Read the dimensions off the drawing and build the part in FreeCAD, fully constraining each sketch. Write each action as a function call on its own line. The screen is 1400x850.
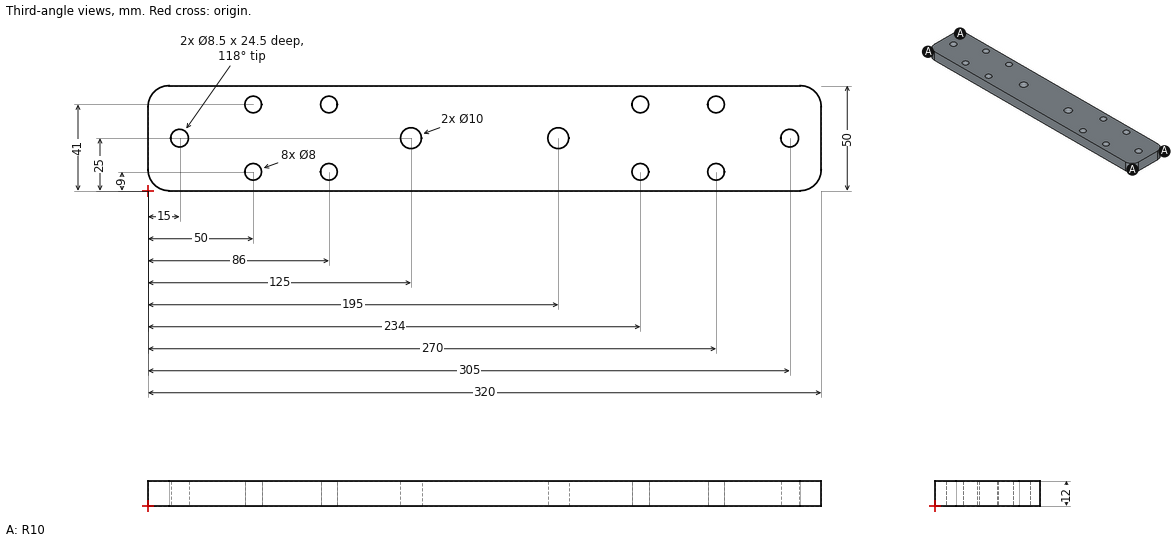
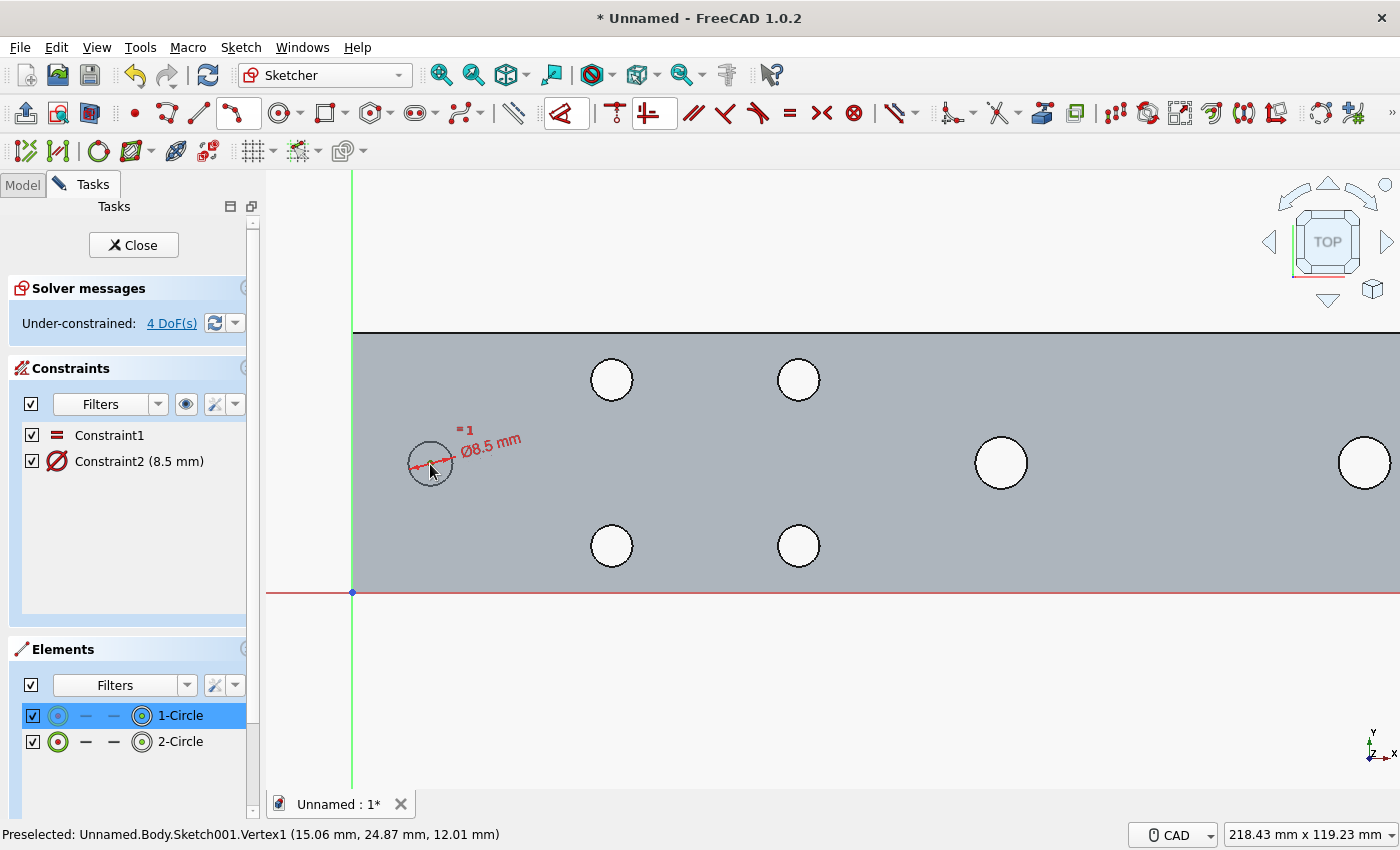
click(584, 114)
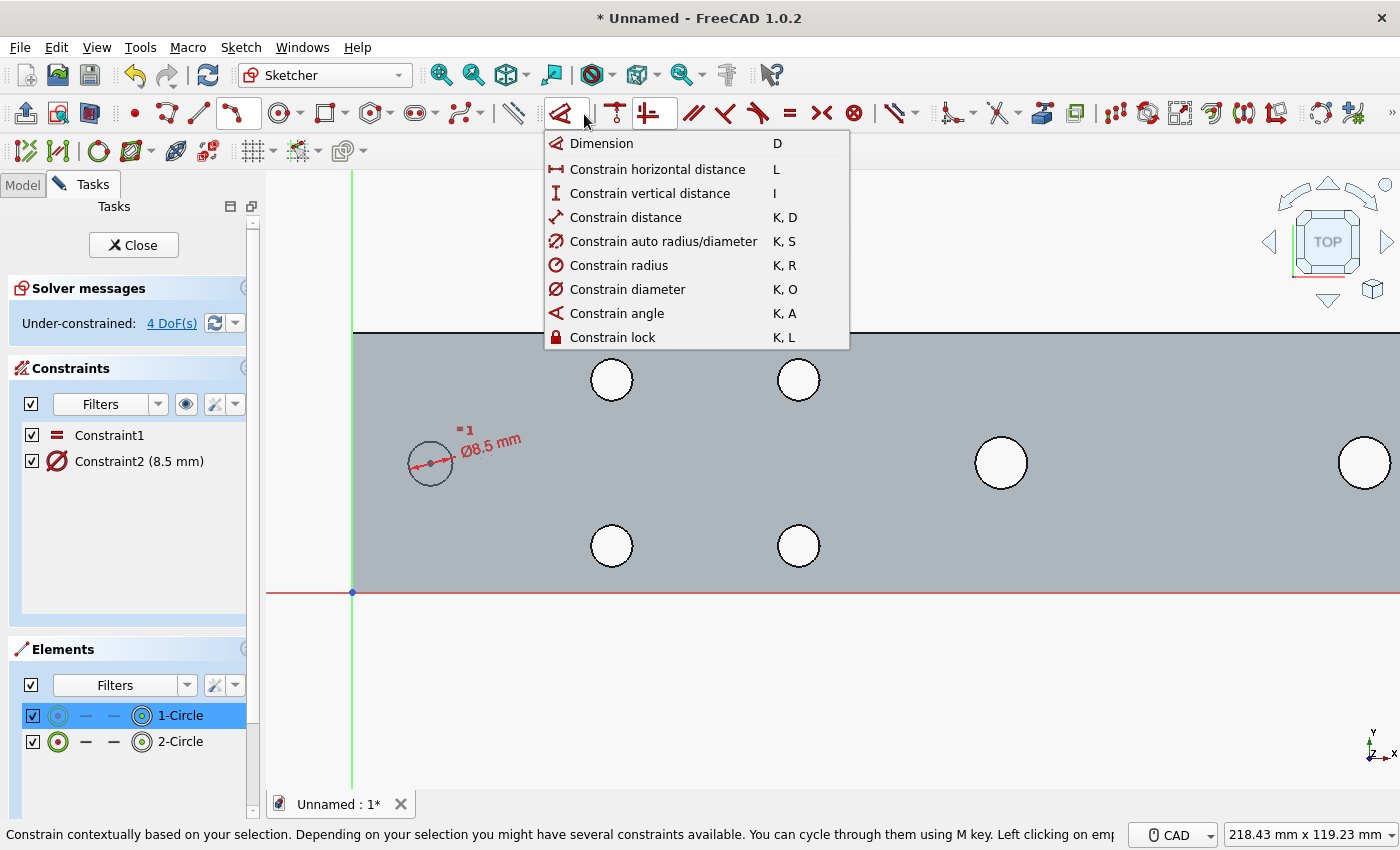
click(697, 169)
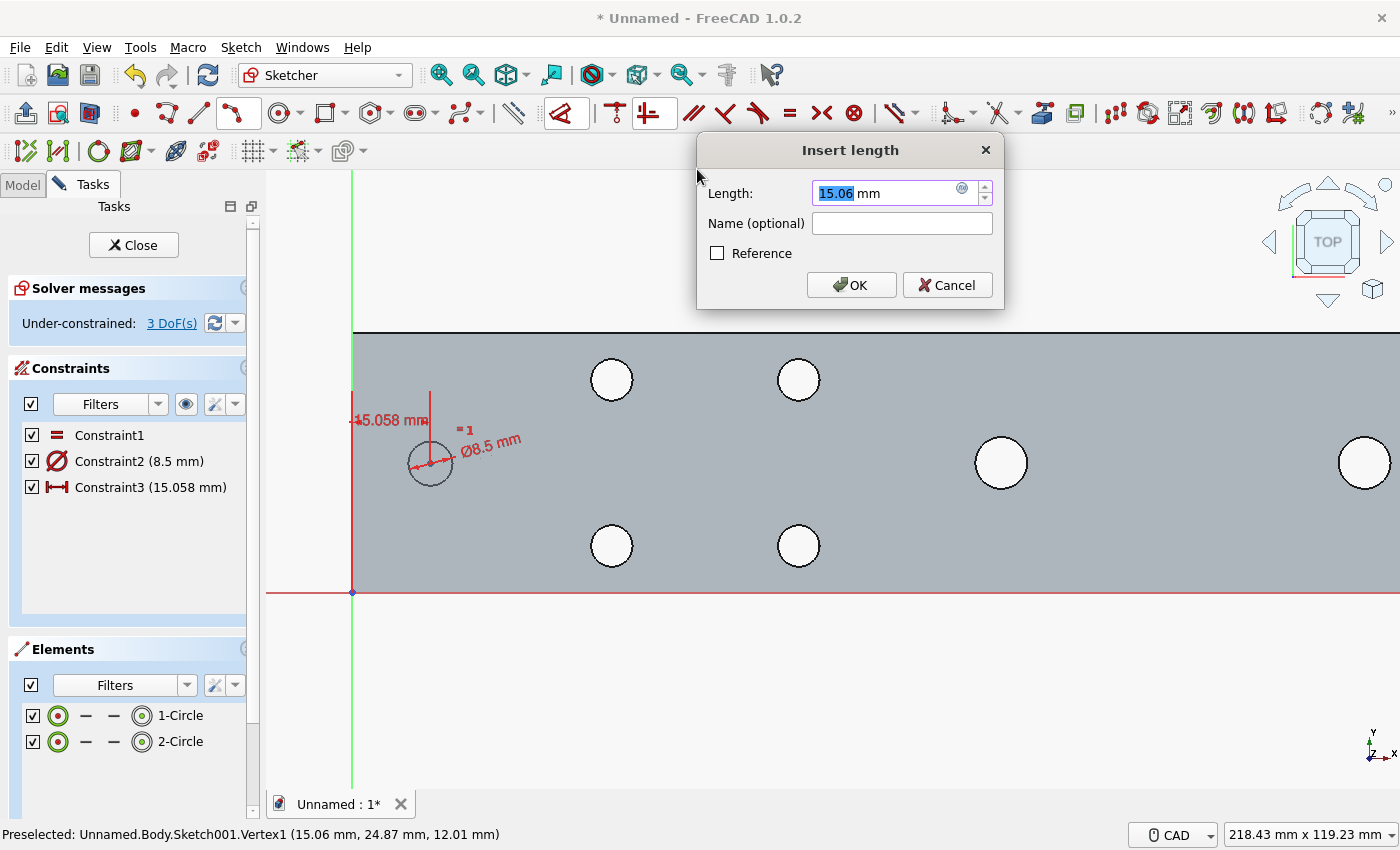
text(15)
key(Return)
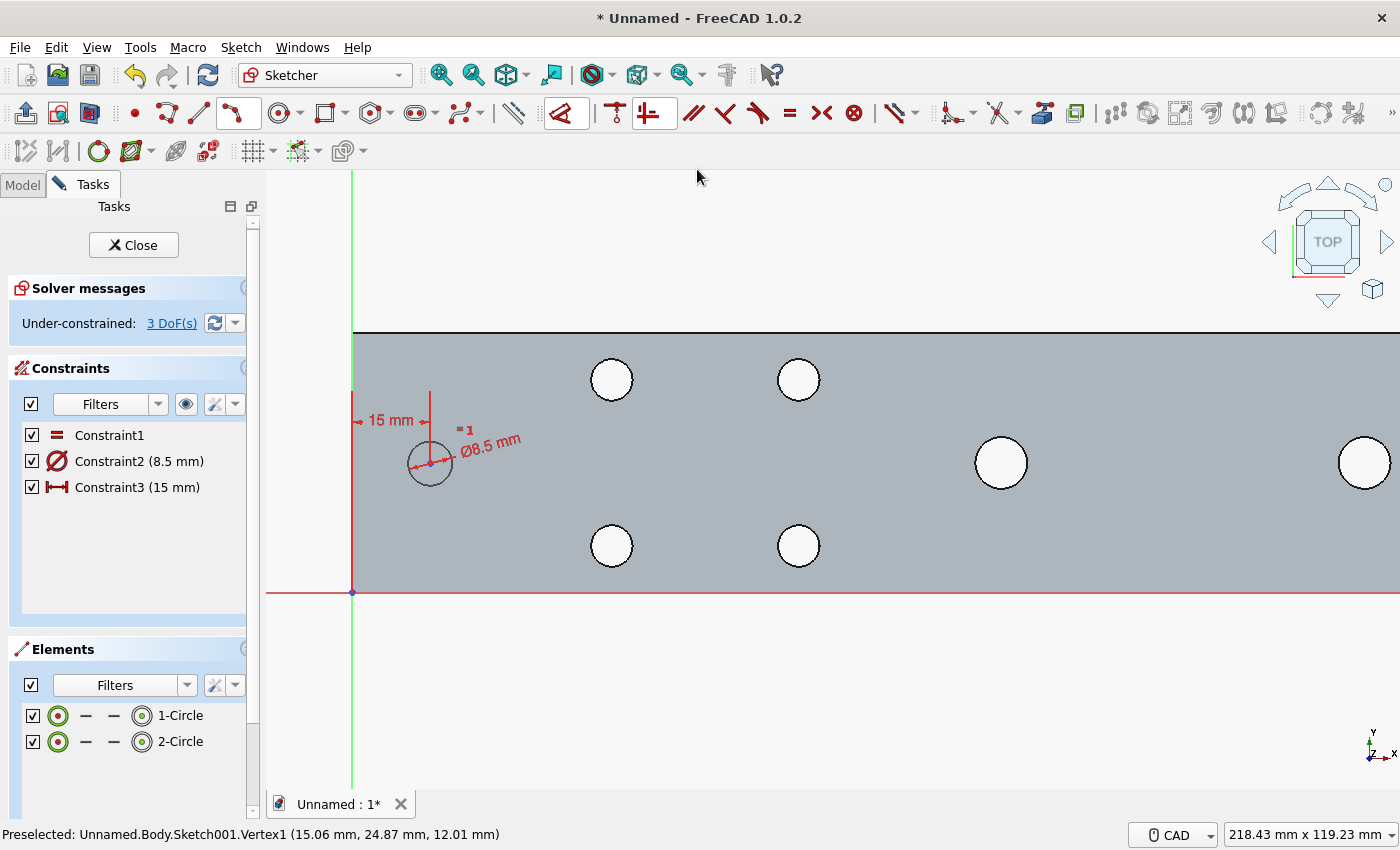
click(430, 464)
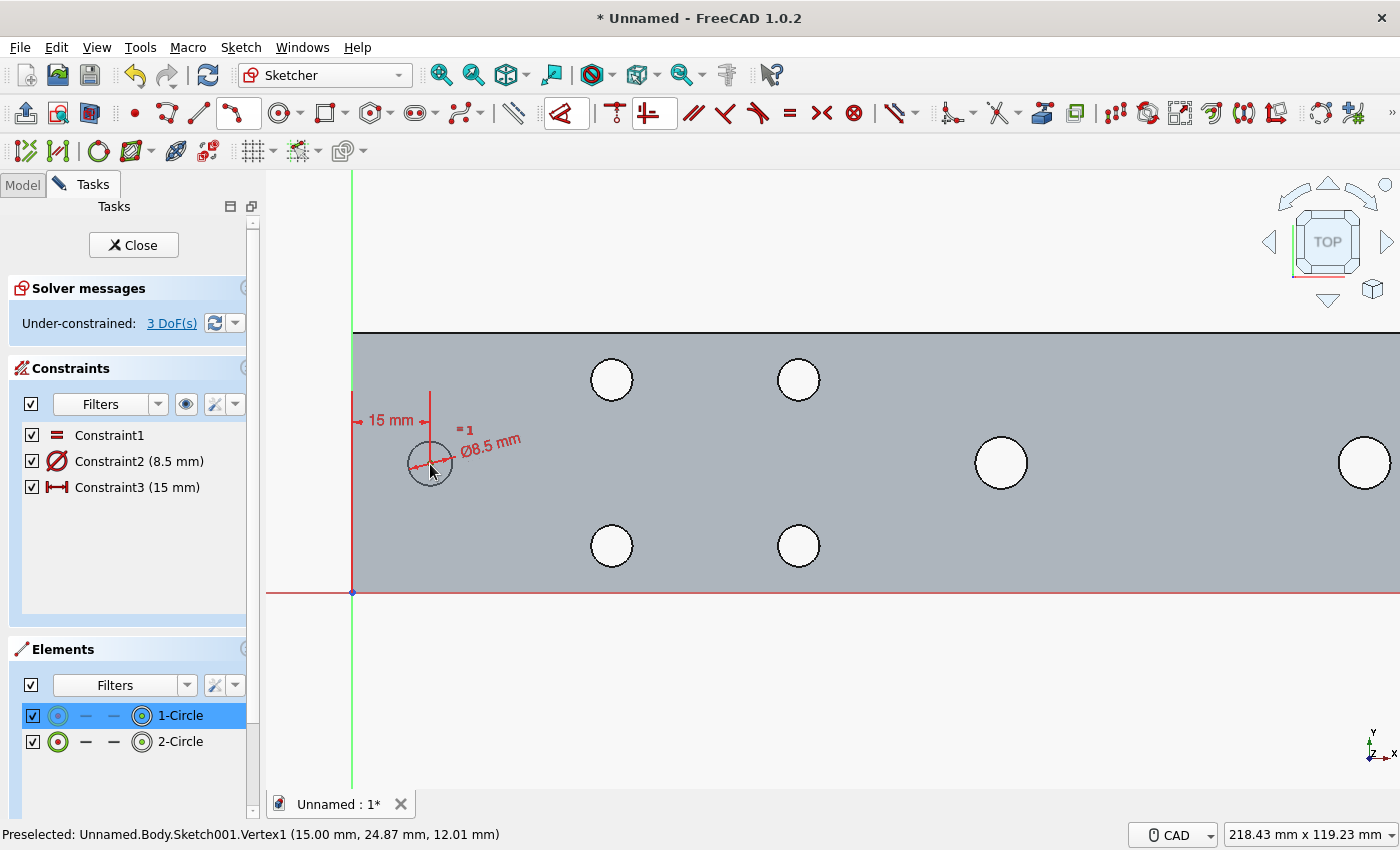
click(584, 114)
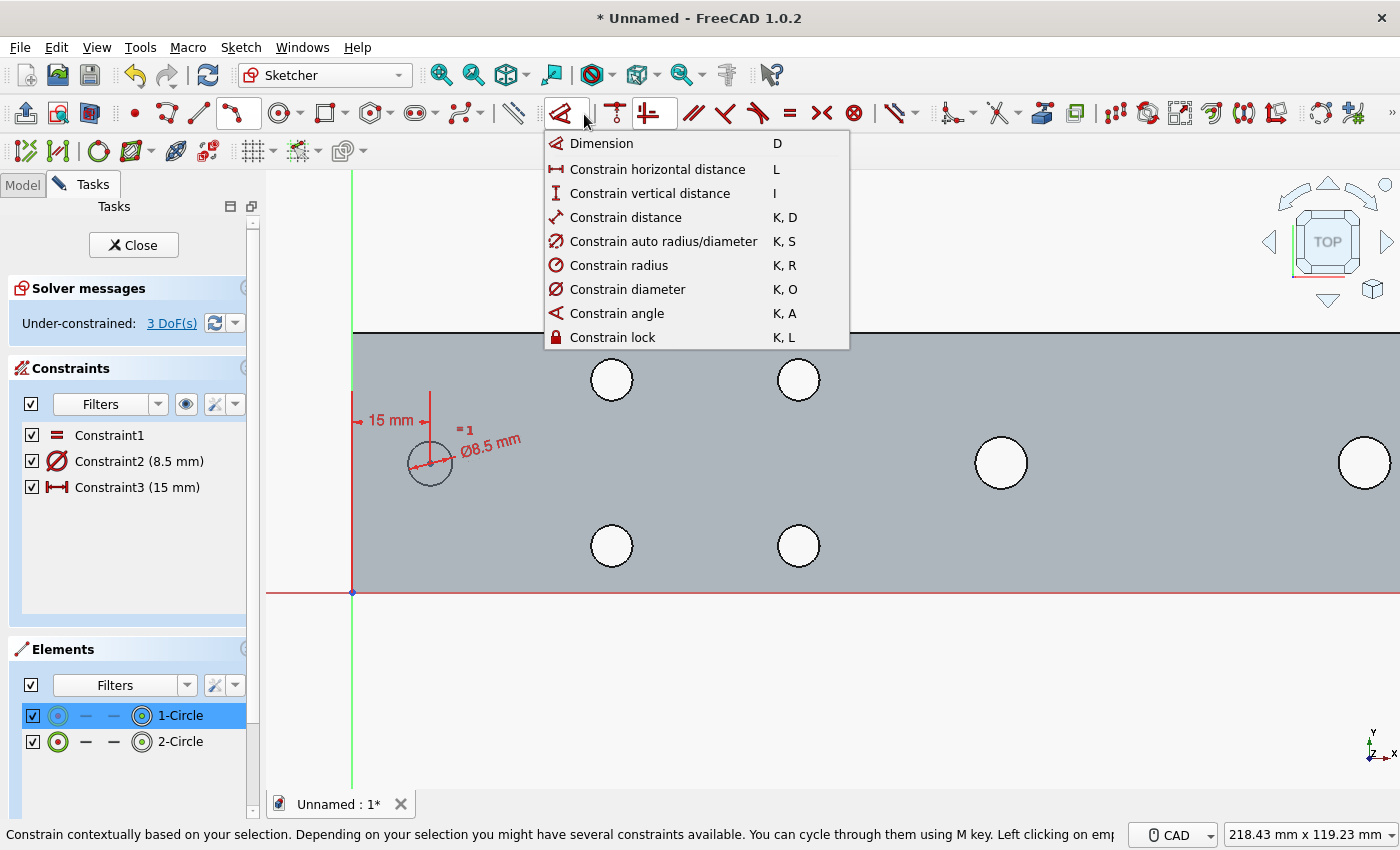
click(697, 193)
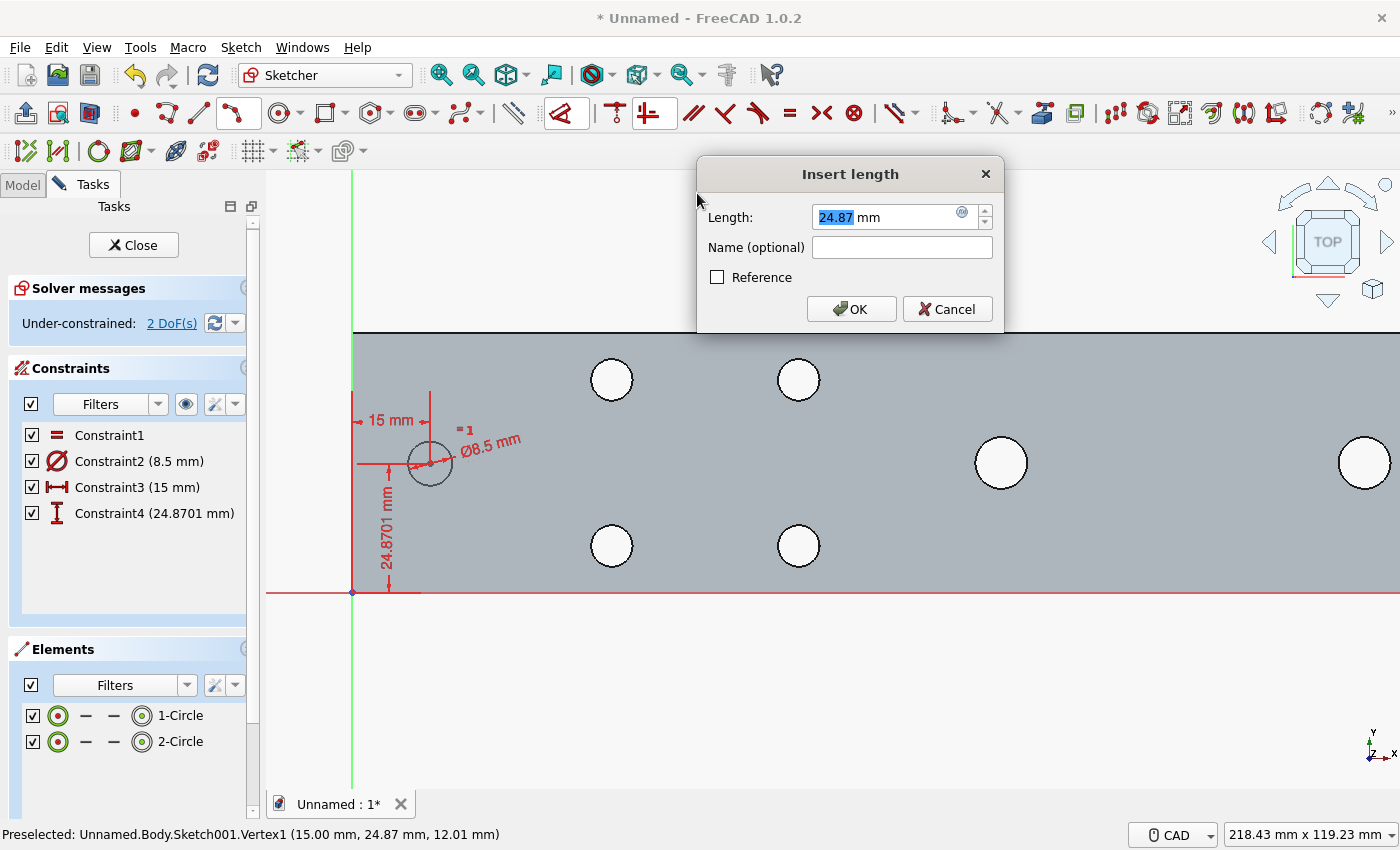
text(25)
key(Return)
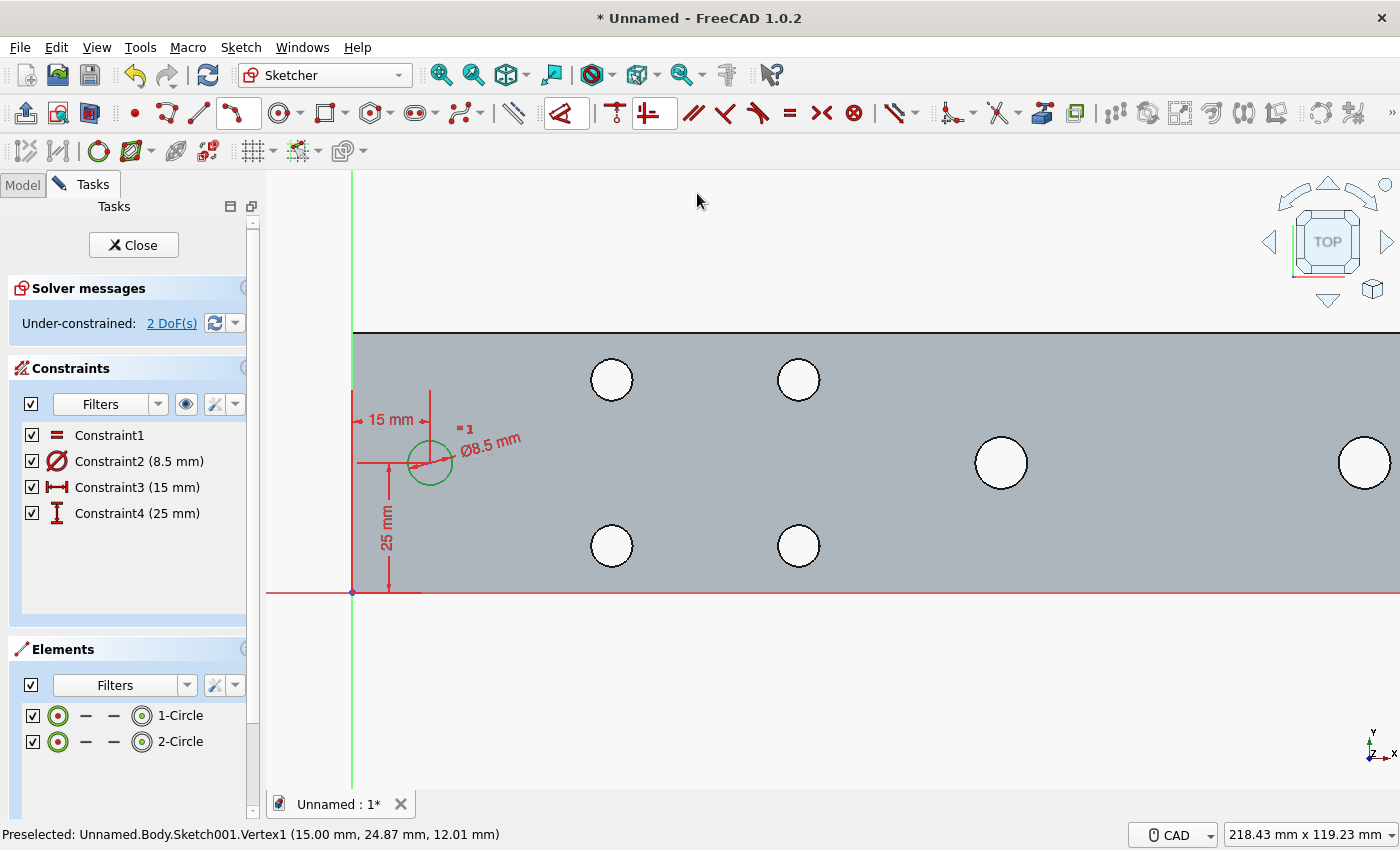
scroll(446, 449, down, 4)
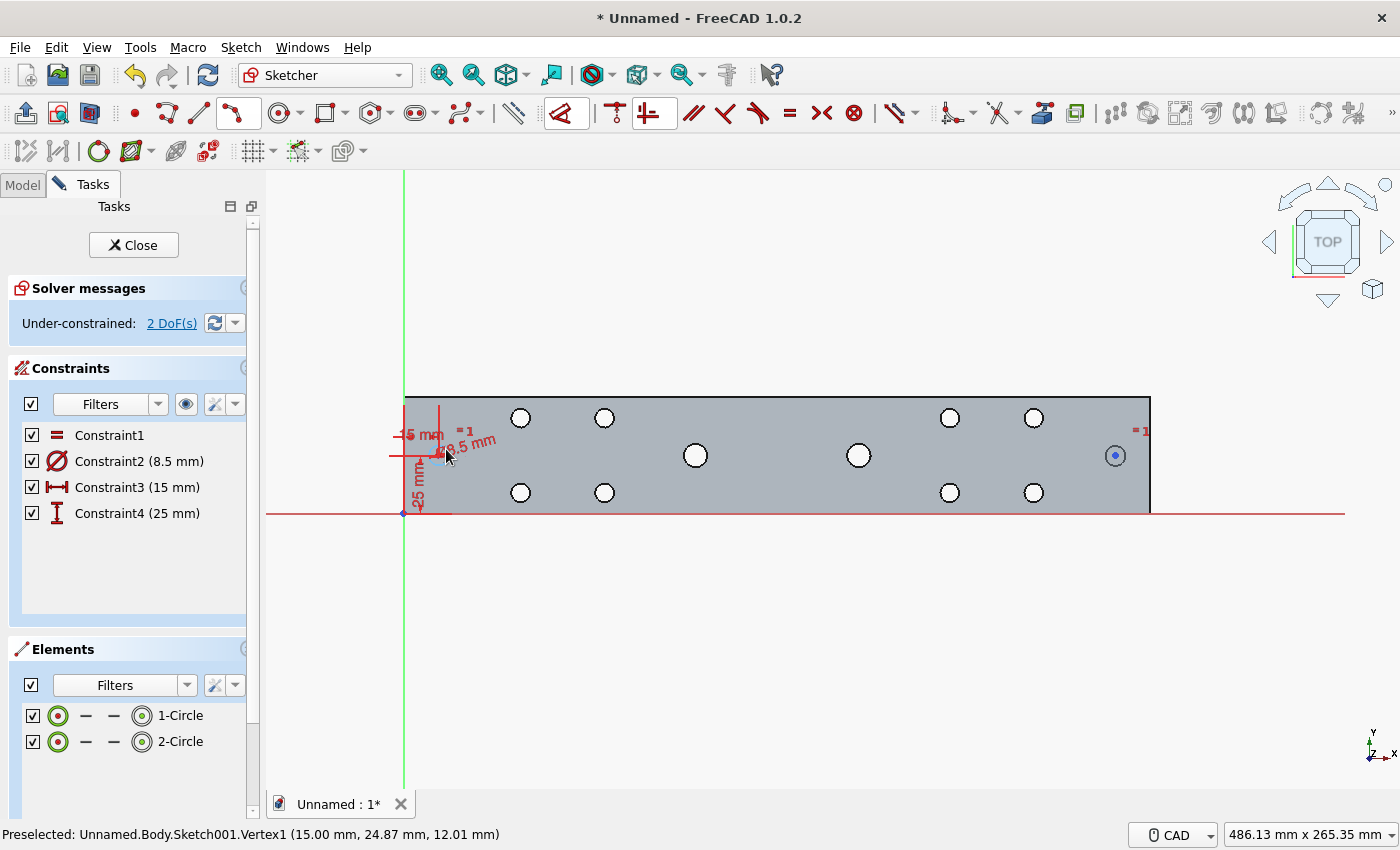
click(1115, 456)